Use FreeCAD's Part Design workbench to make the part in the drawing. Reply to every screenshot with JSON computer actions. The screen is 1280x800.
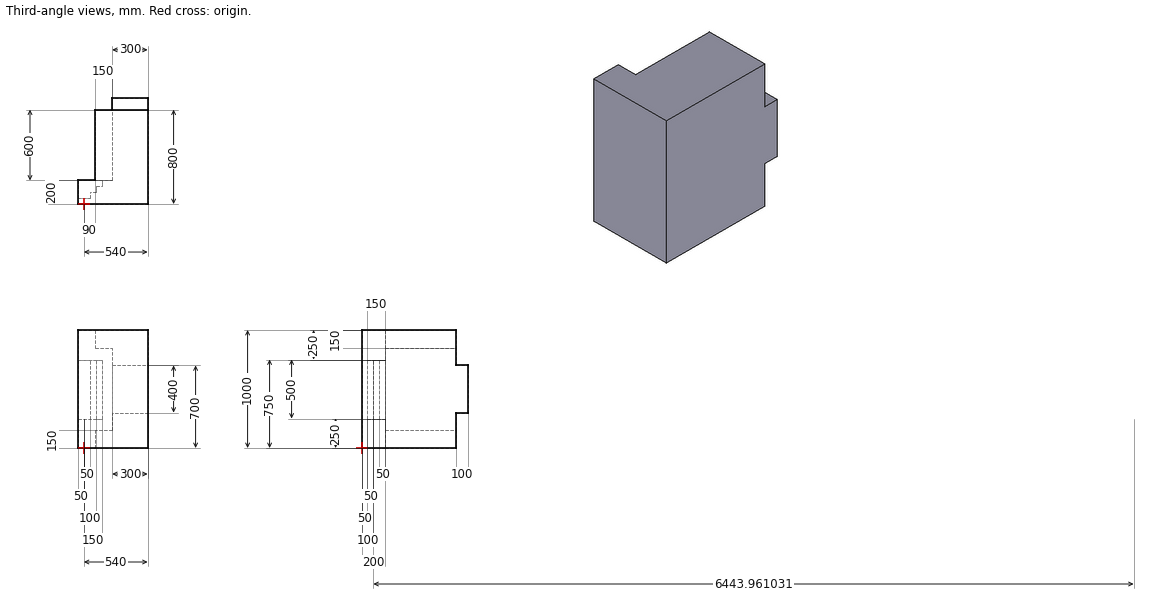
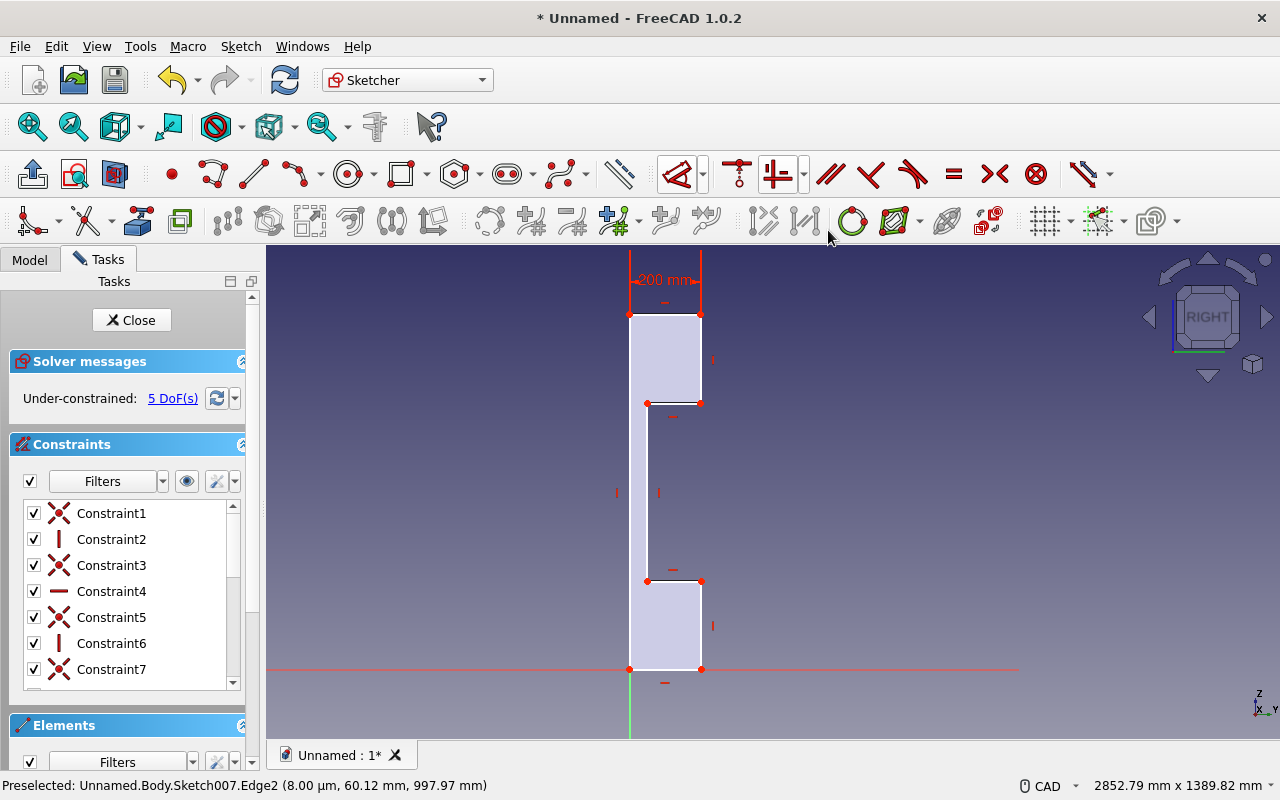
{"action": "left_click", "coordinate": [701, 342]}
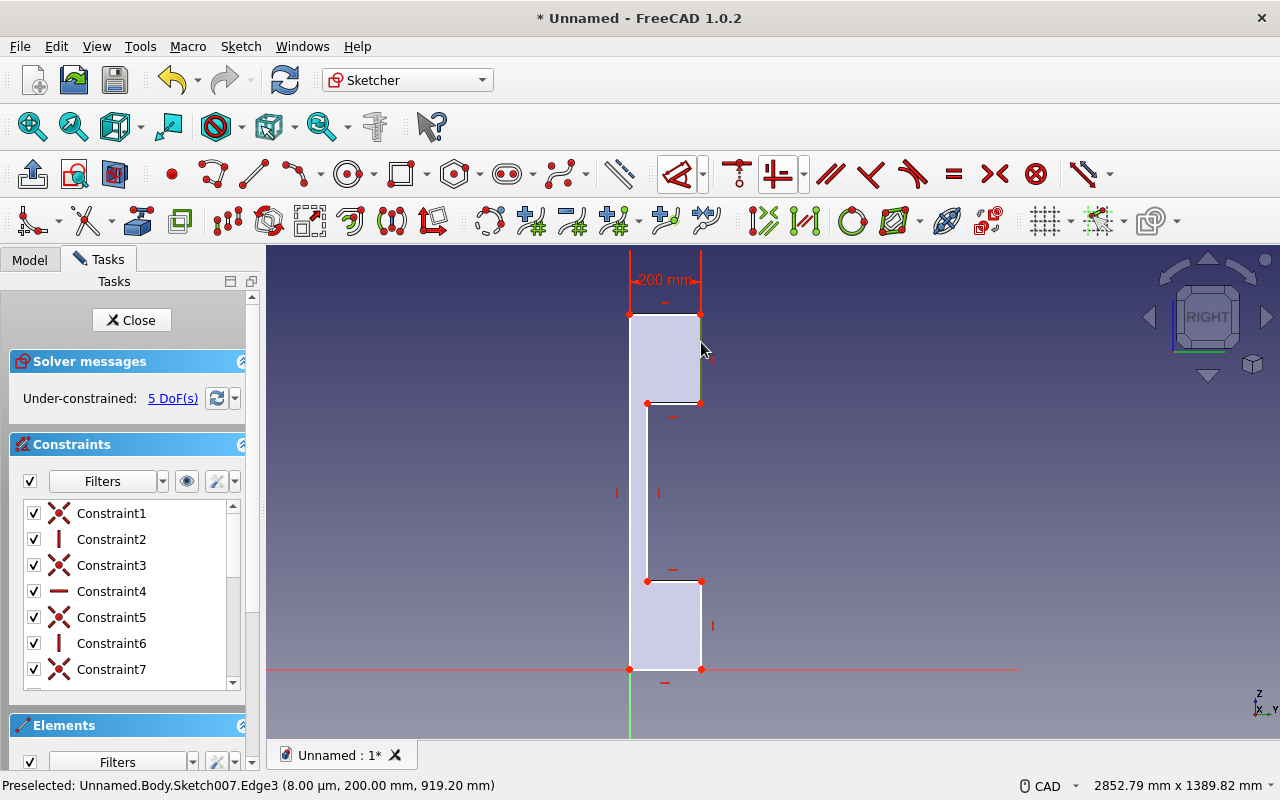
{"action": "left_click", "coordinate": [702, 174]}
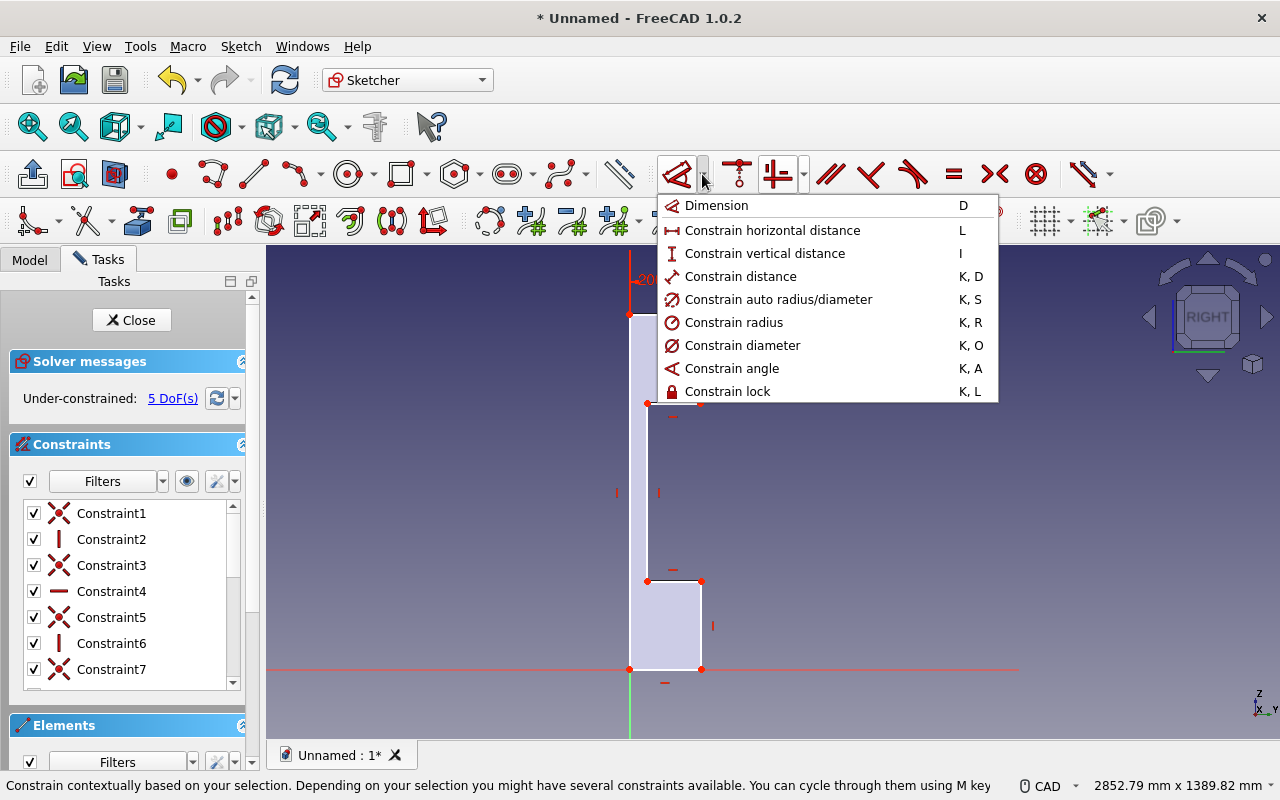
{"action": "left_click", "coordinate": [828, 254]}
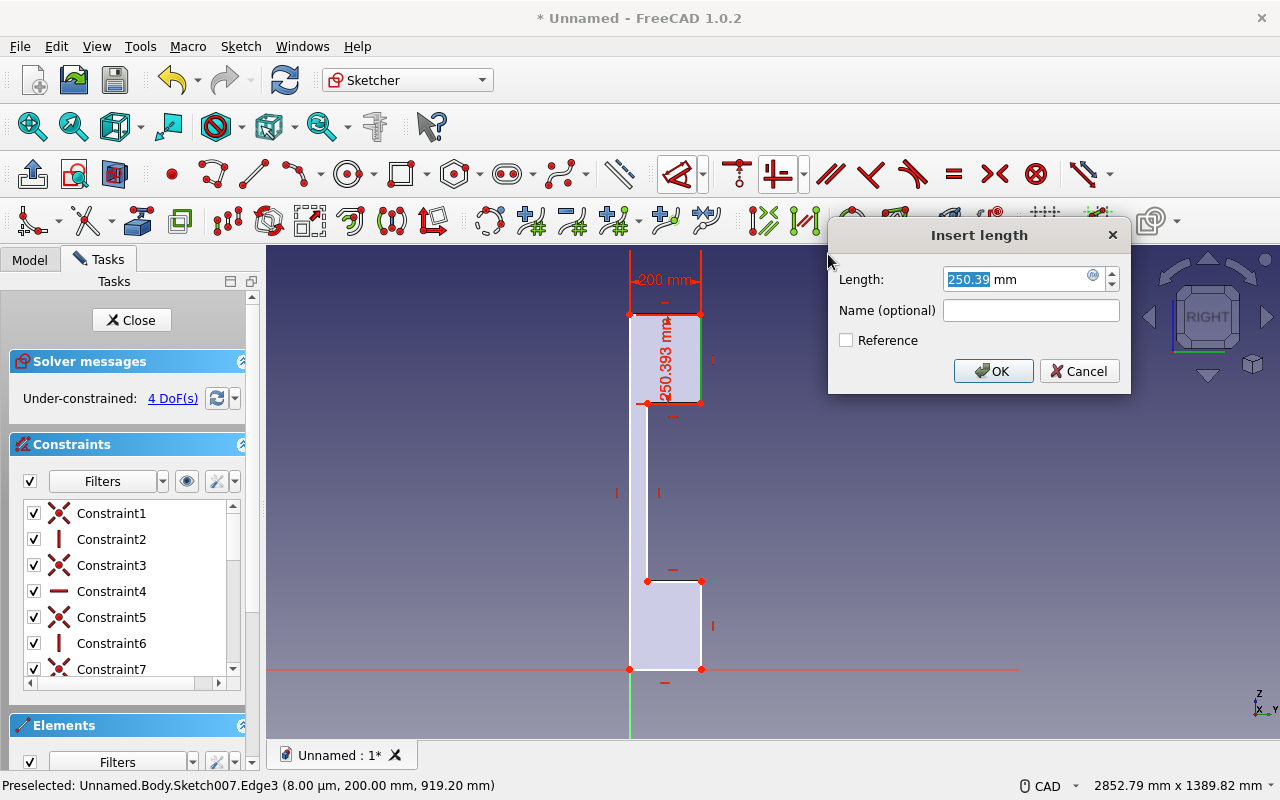
{"action": "type", "text": "250"}
{"action": "key", "text": "Return"}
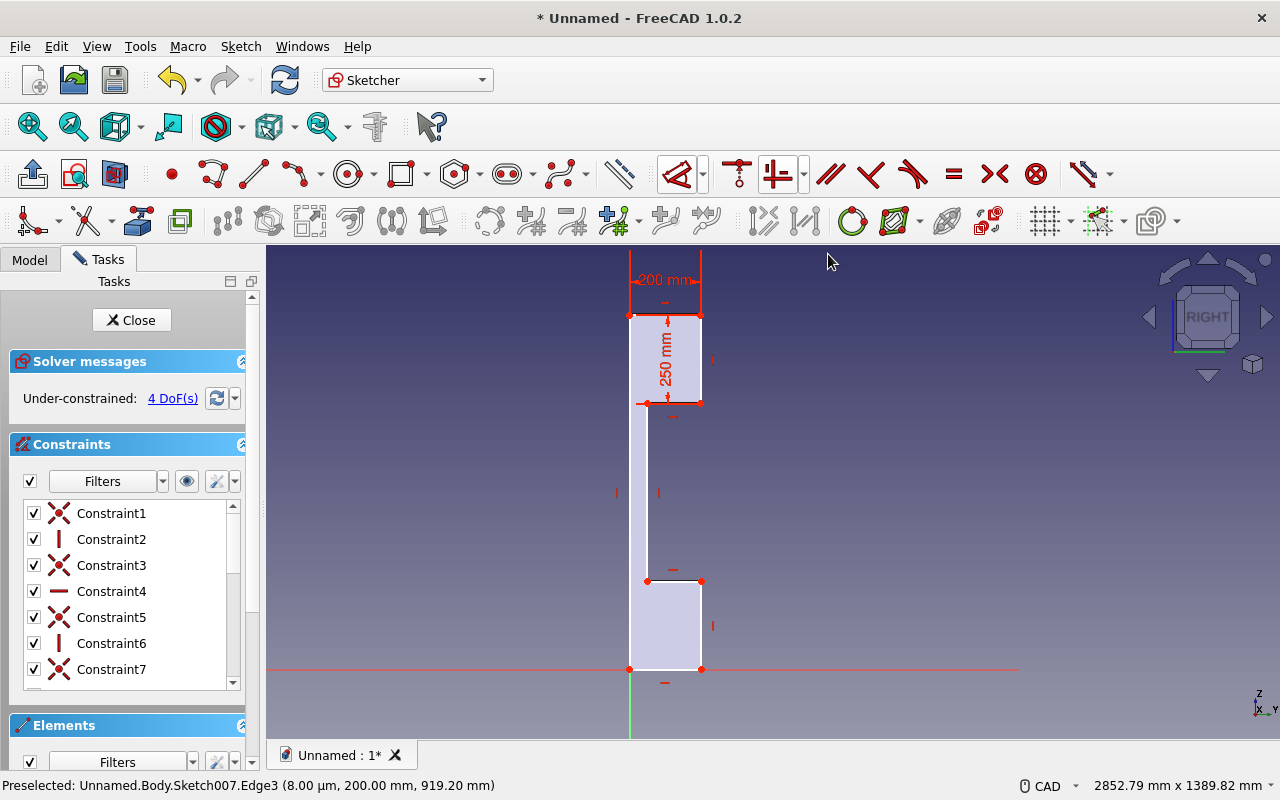
{"action": "left_click", "coordinate": [685, 404]}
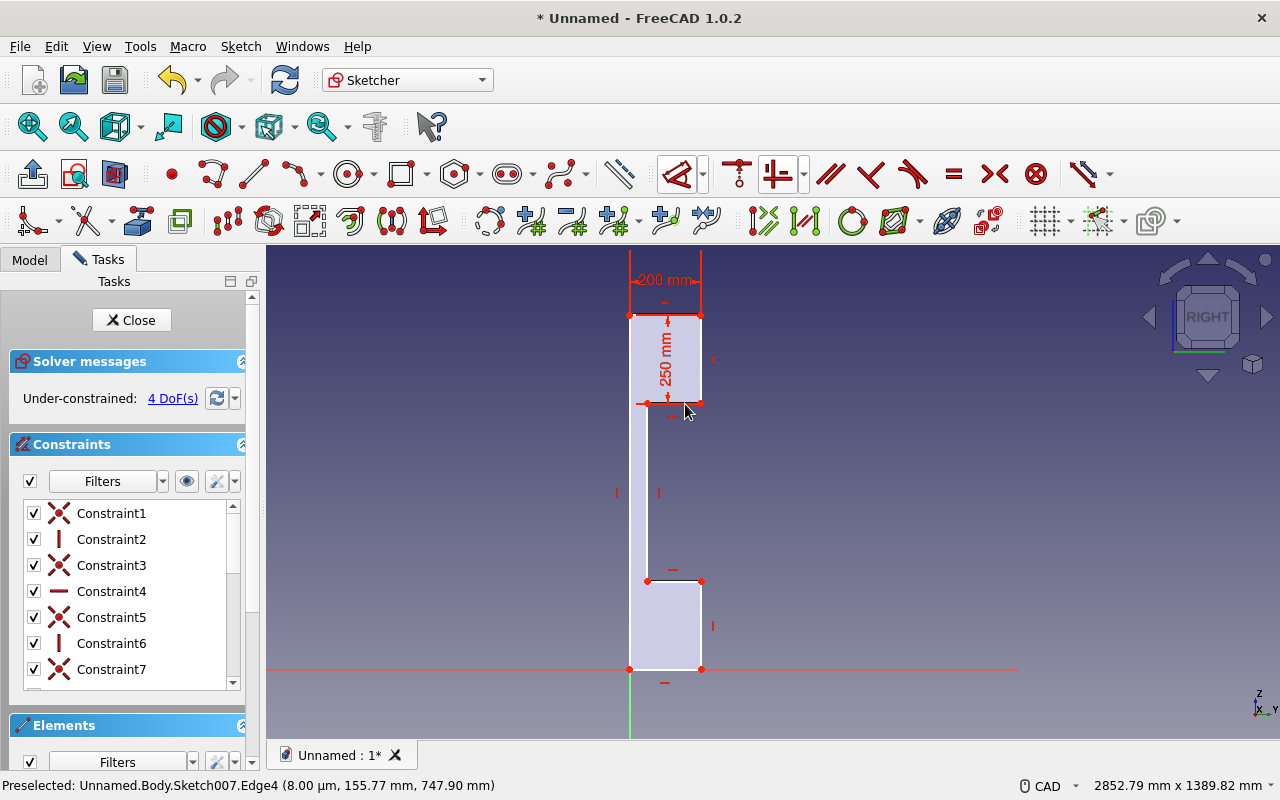
{"action": "key", "text": "l"}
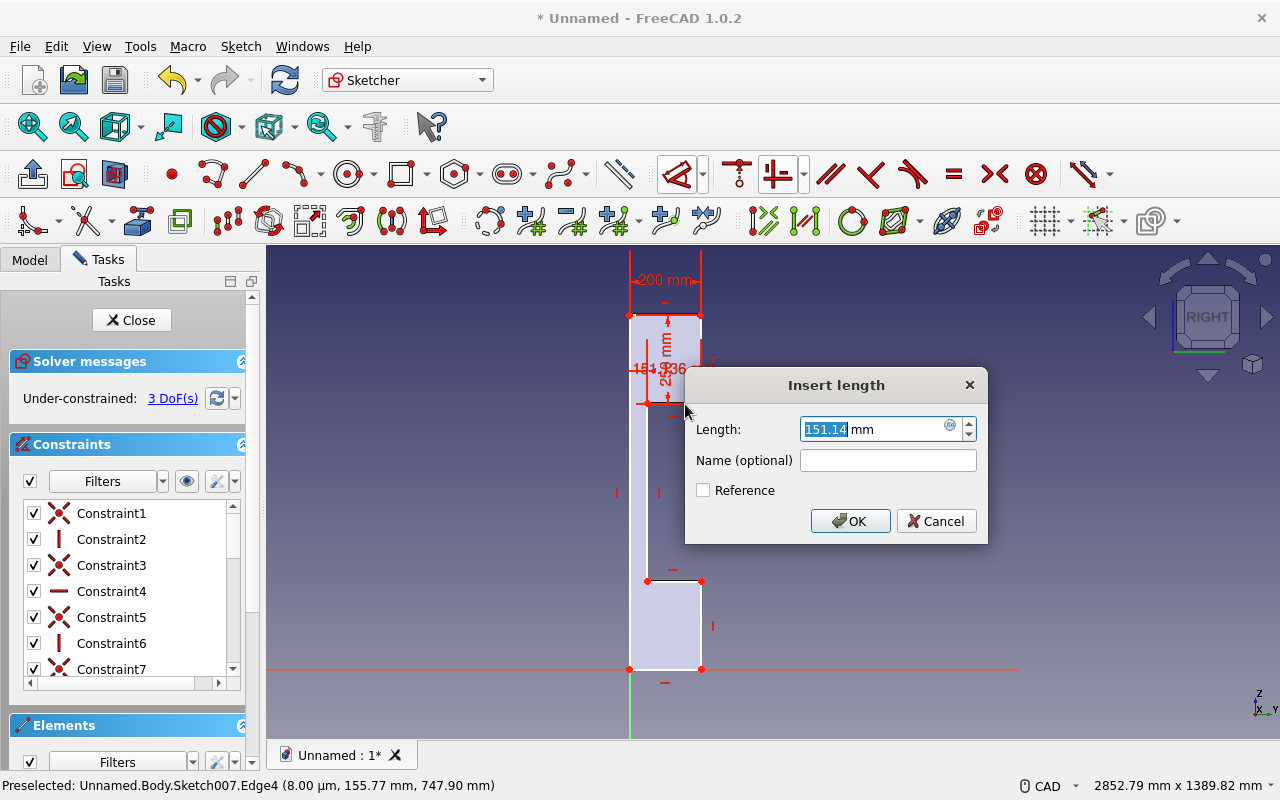
{"action": "type", "text": "150"}
{"action": "key", "text": "Return"}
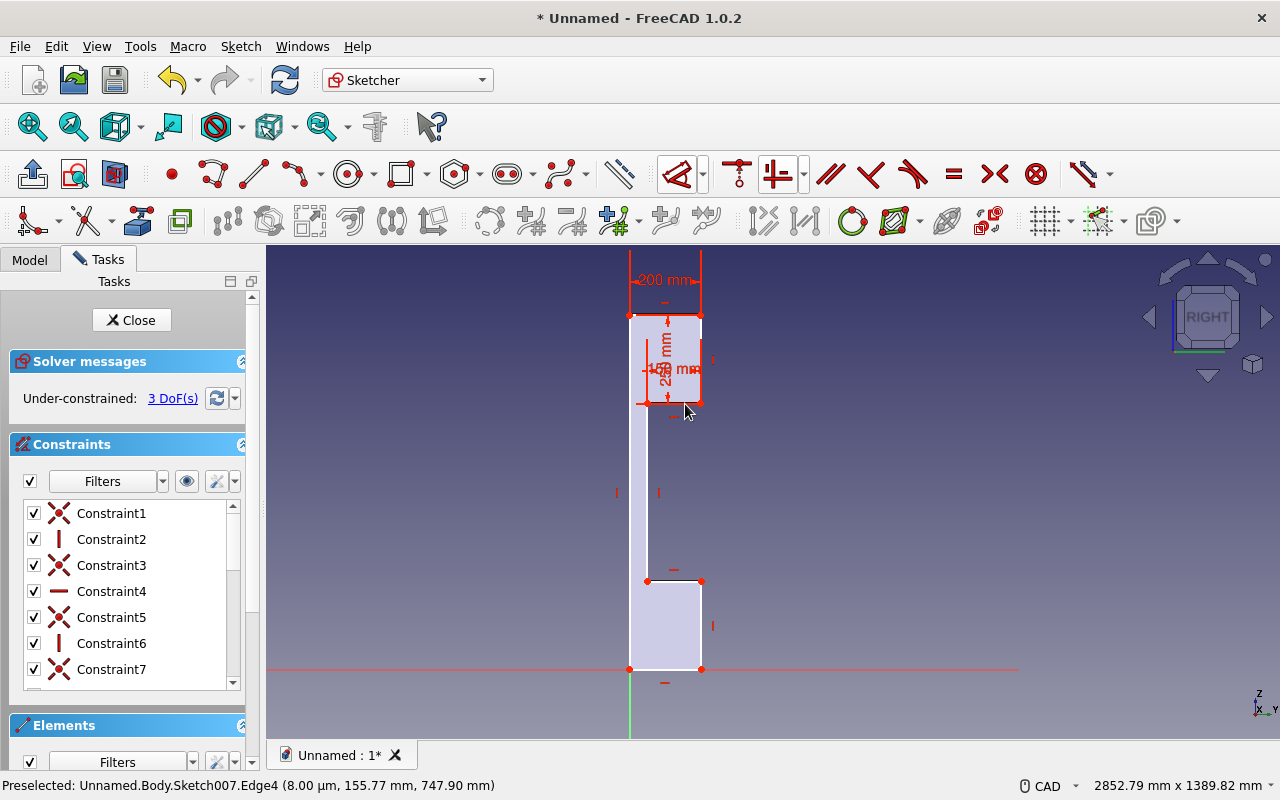
{"action": "left_click", "coordinate": [647, 457]}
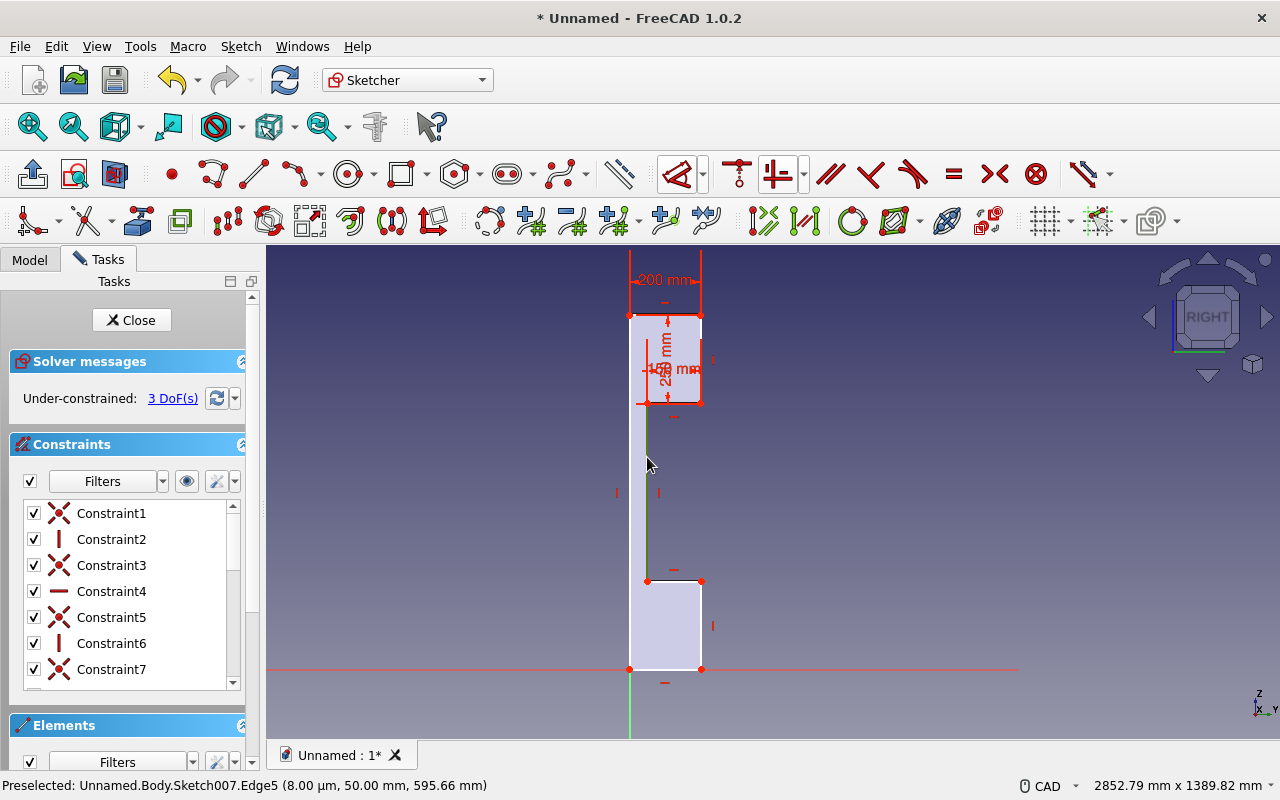
{"action": "left_click", "coordinate": [702, 174]}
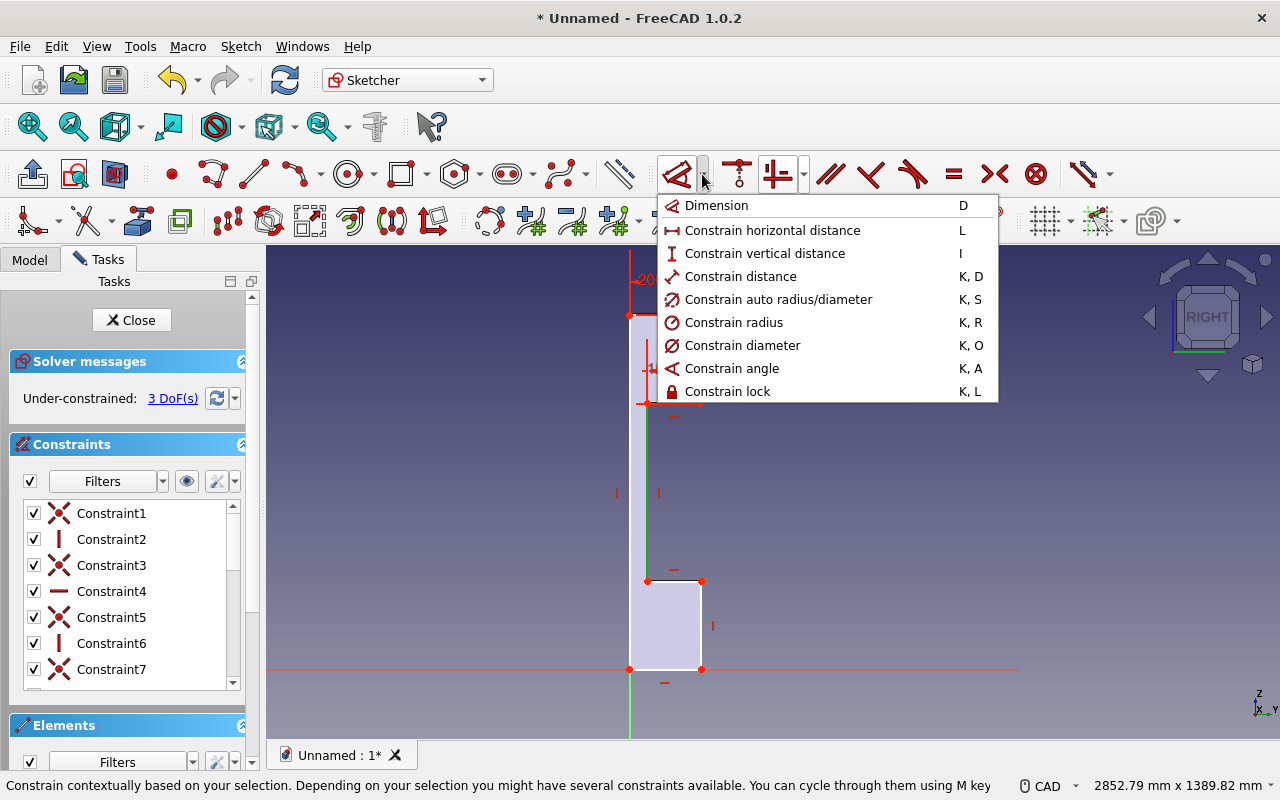
{"action": "left_click", "coordinate": [828, 254]}